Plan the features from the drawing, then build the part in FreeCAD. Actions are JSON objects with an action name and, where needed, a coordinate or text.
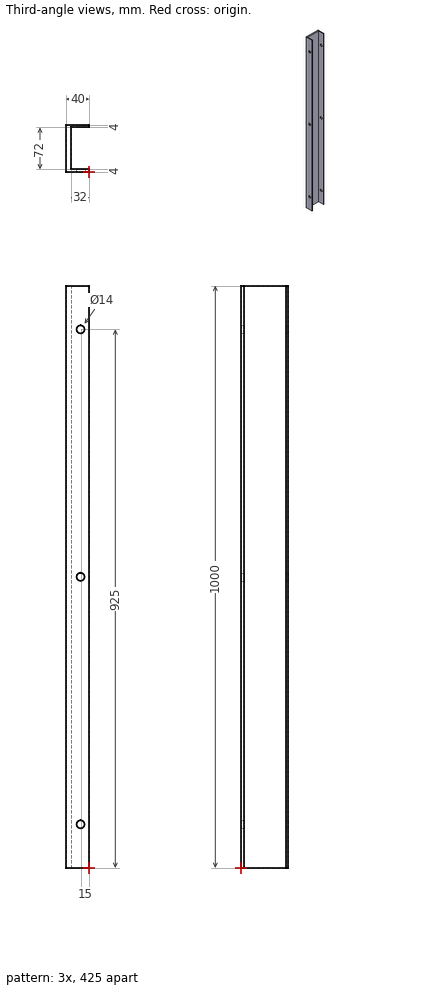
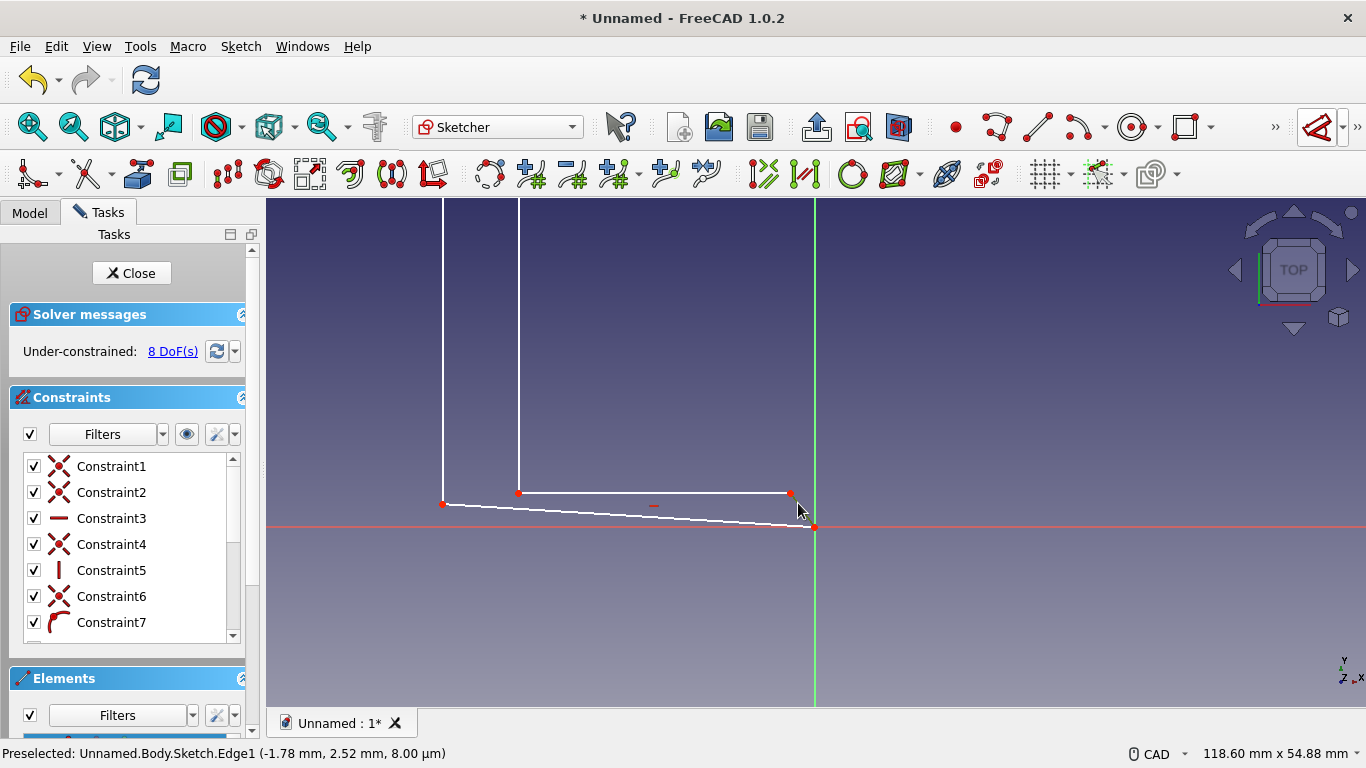
{"action": "key", "text": "v"}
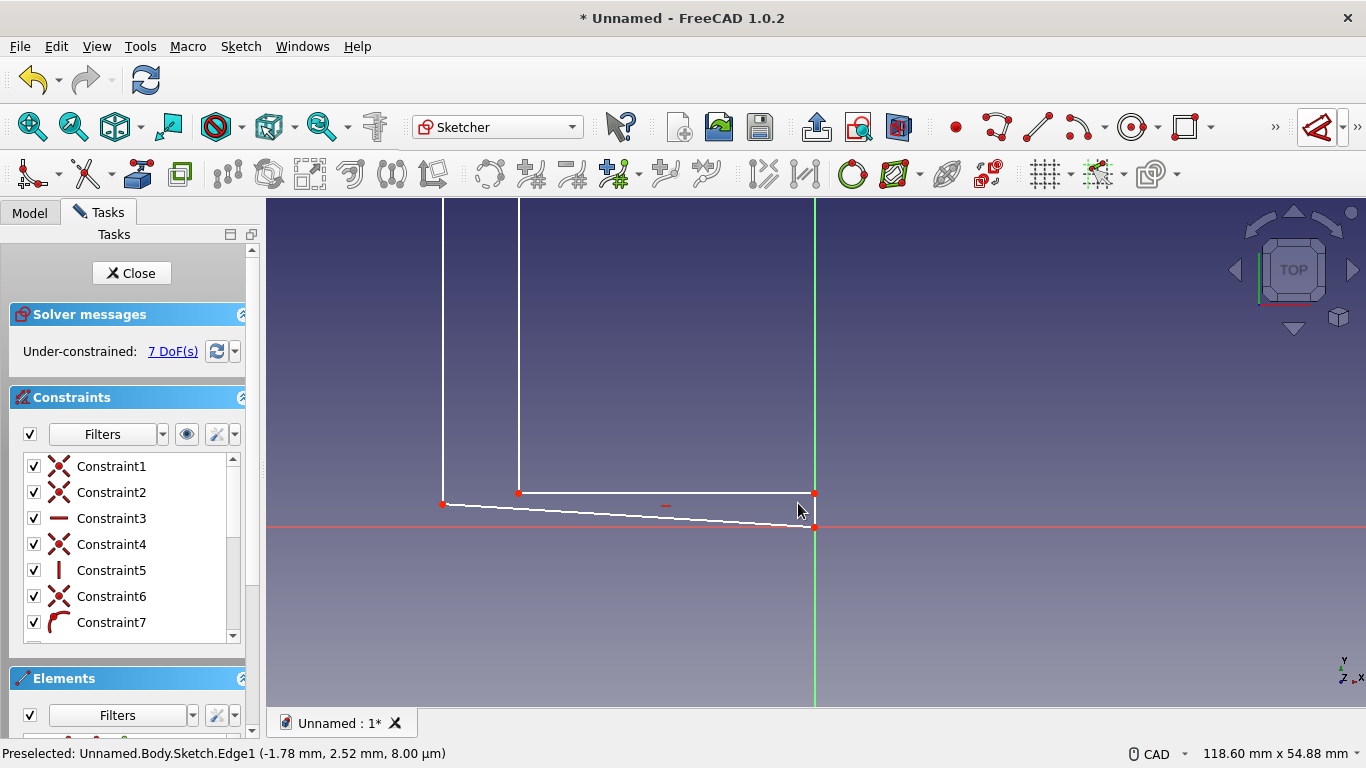
{"action": "scroll", "coordinate": [844, 679], "scroll_direction": "down", "scroll_amount": 4}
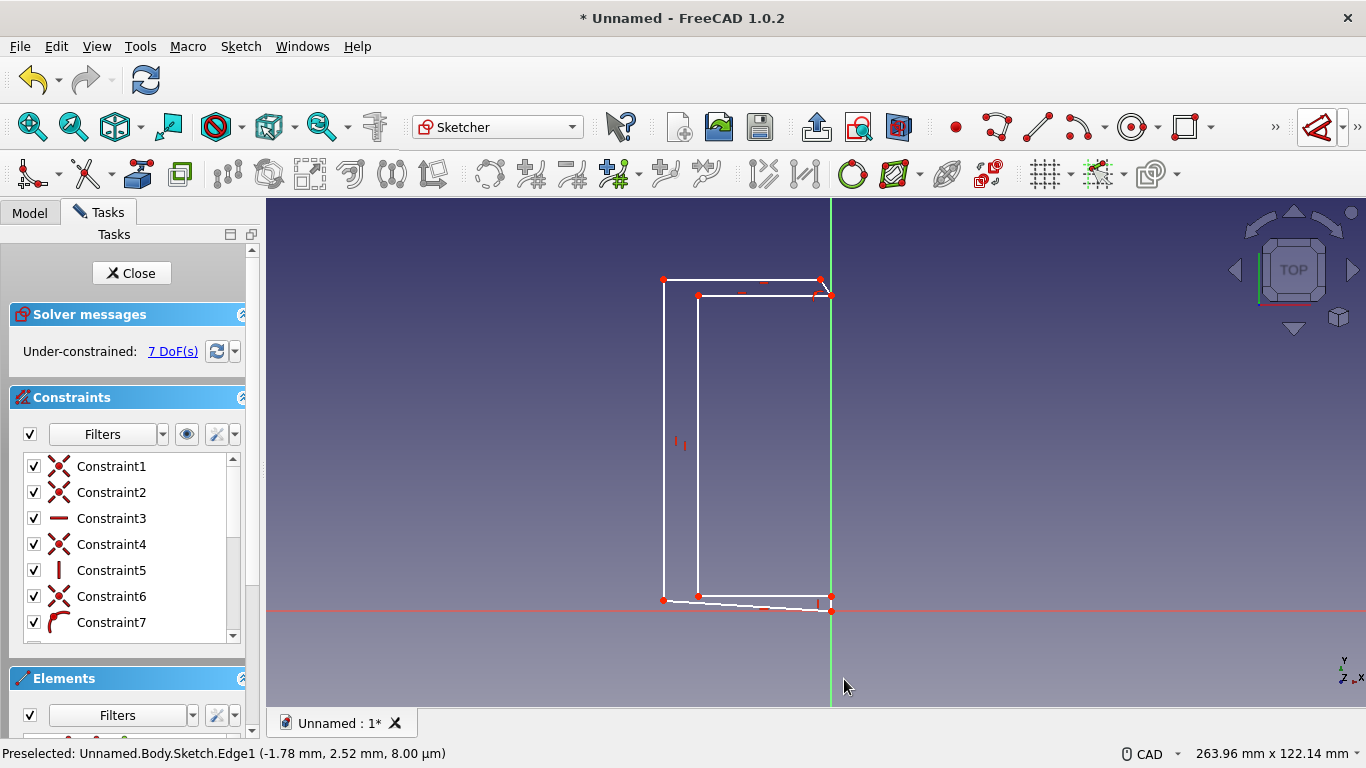
{"action": "scroll", "coordinate": [824, 284], "scroll_direction": "up", "scroll_amount": 5}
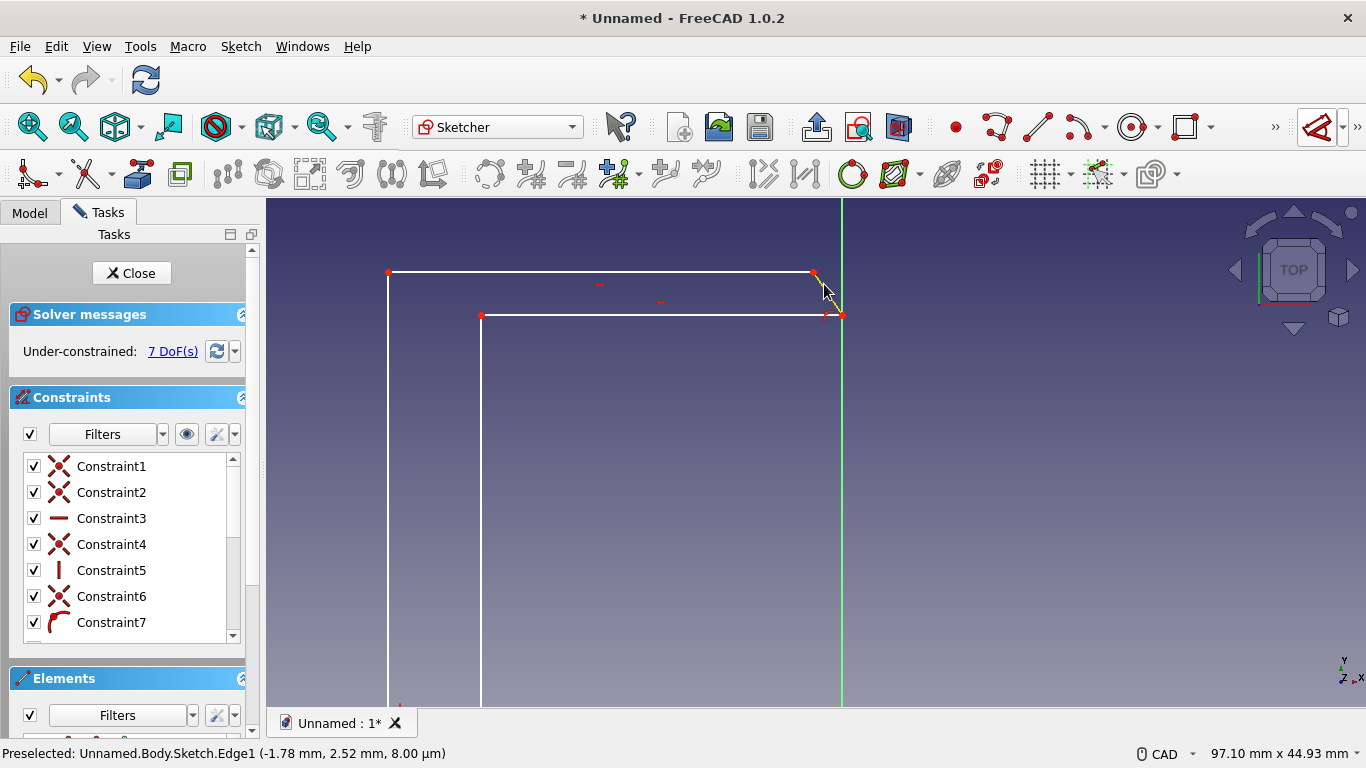
{"action": "left_click", "coordinate": [822, 285]}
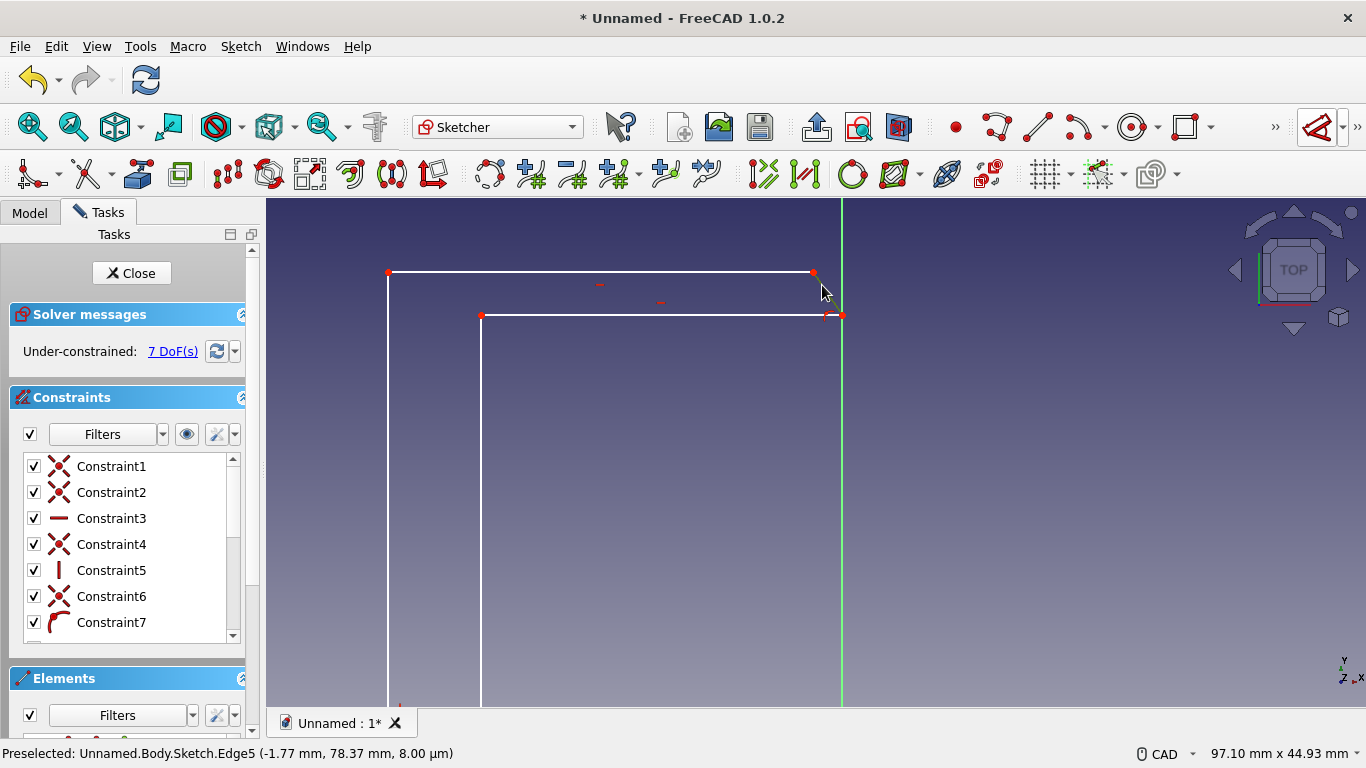
{"action": "key", "text": "v"}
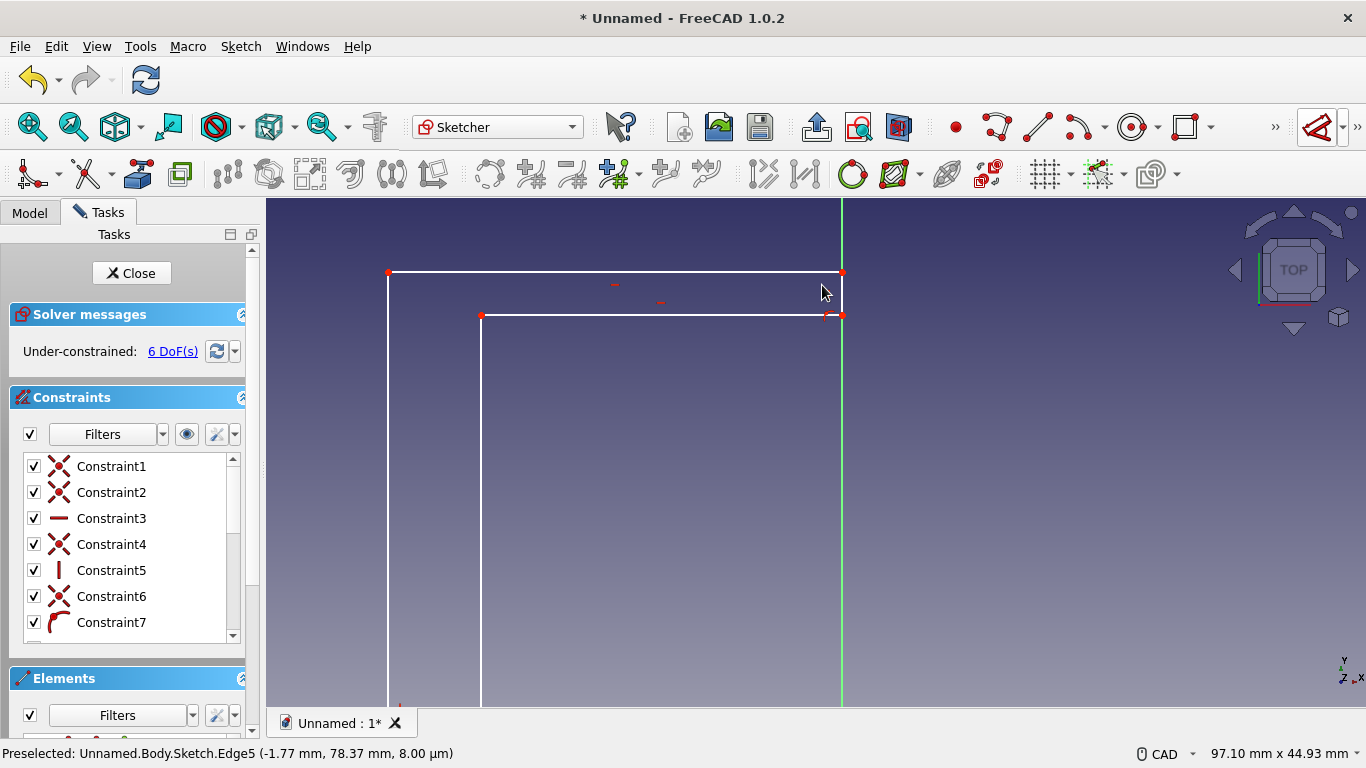
{"action": "scroll", "coordinate": [824, 297], "scroll_direction": "down", "scroll_amount": 5}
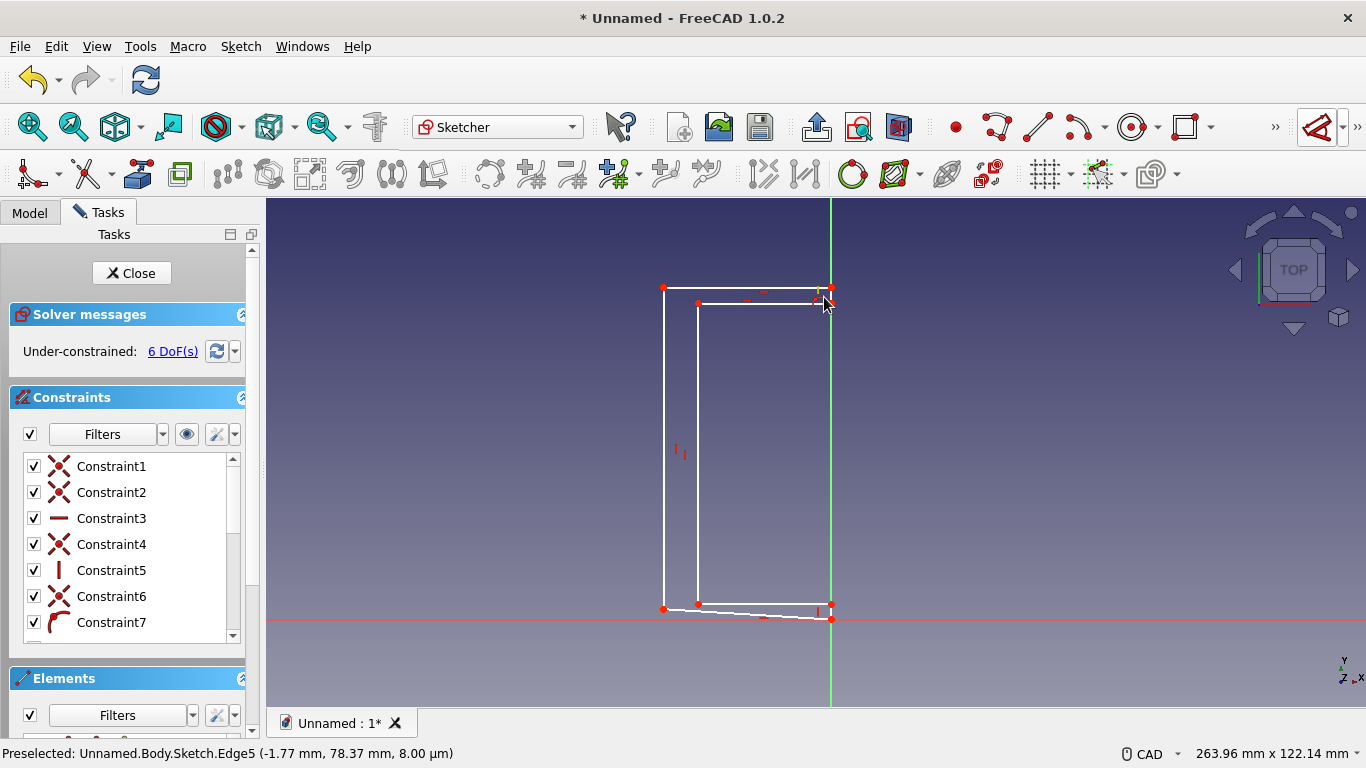
{"action": "scroll", "coordinate": [714, 612], "scroll_direction": "up", "scroll_amount": 4}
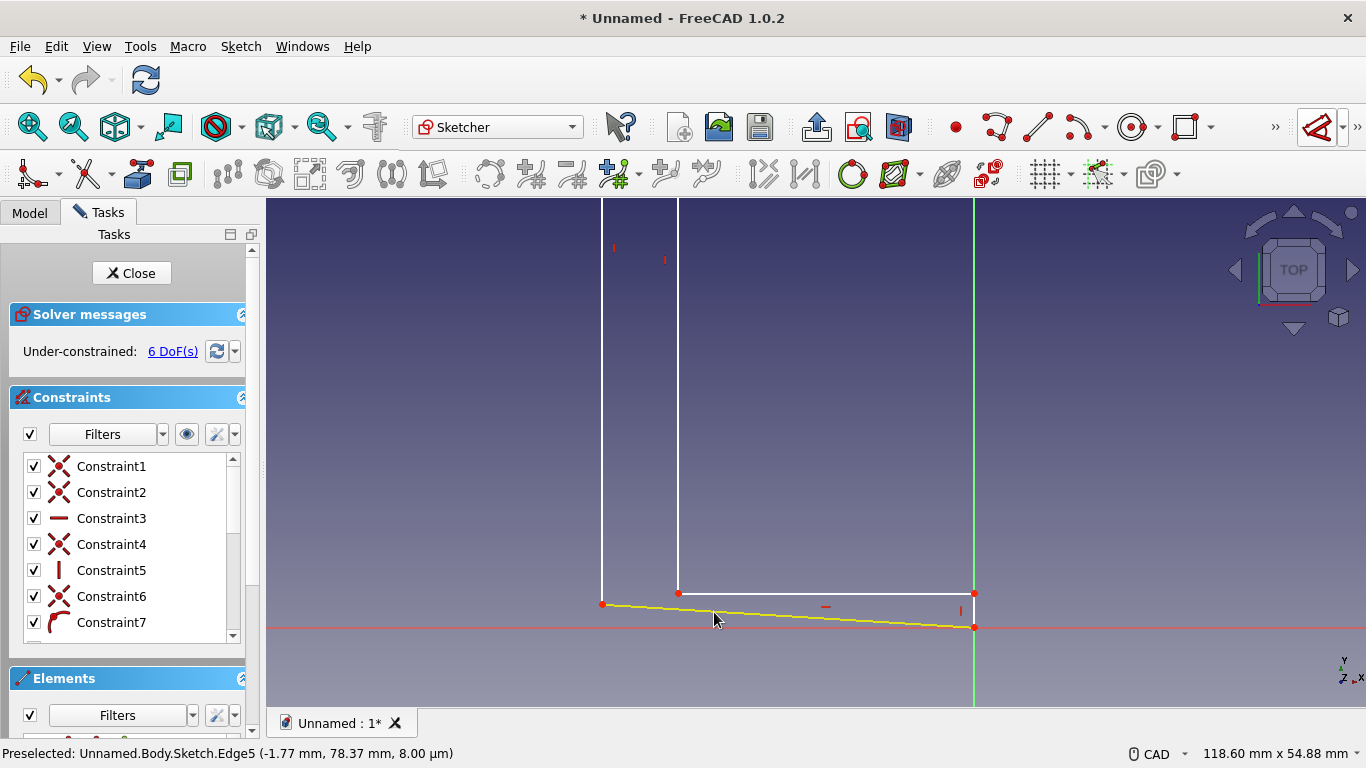
{"action": "left_click", "coordinate": [714, 612]}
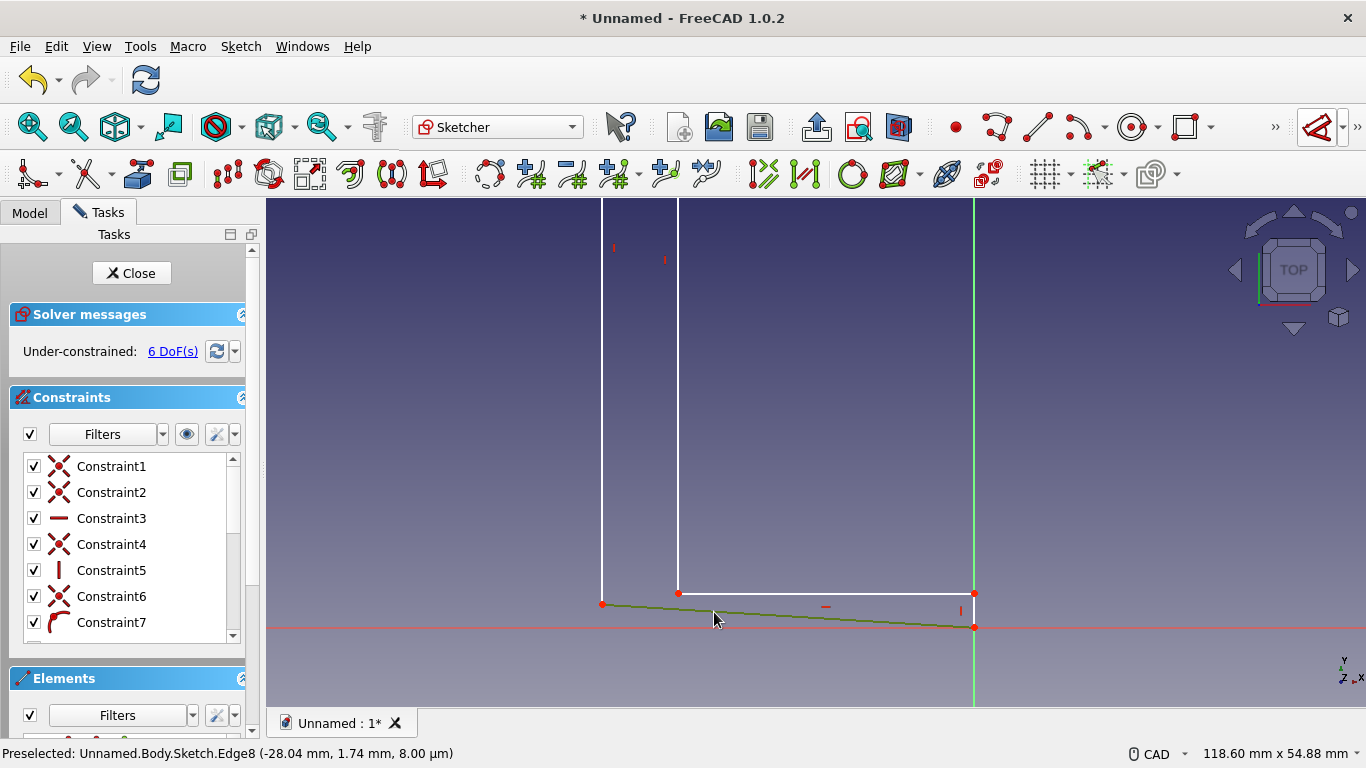
{"action": "key", "text": "h"}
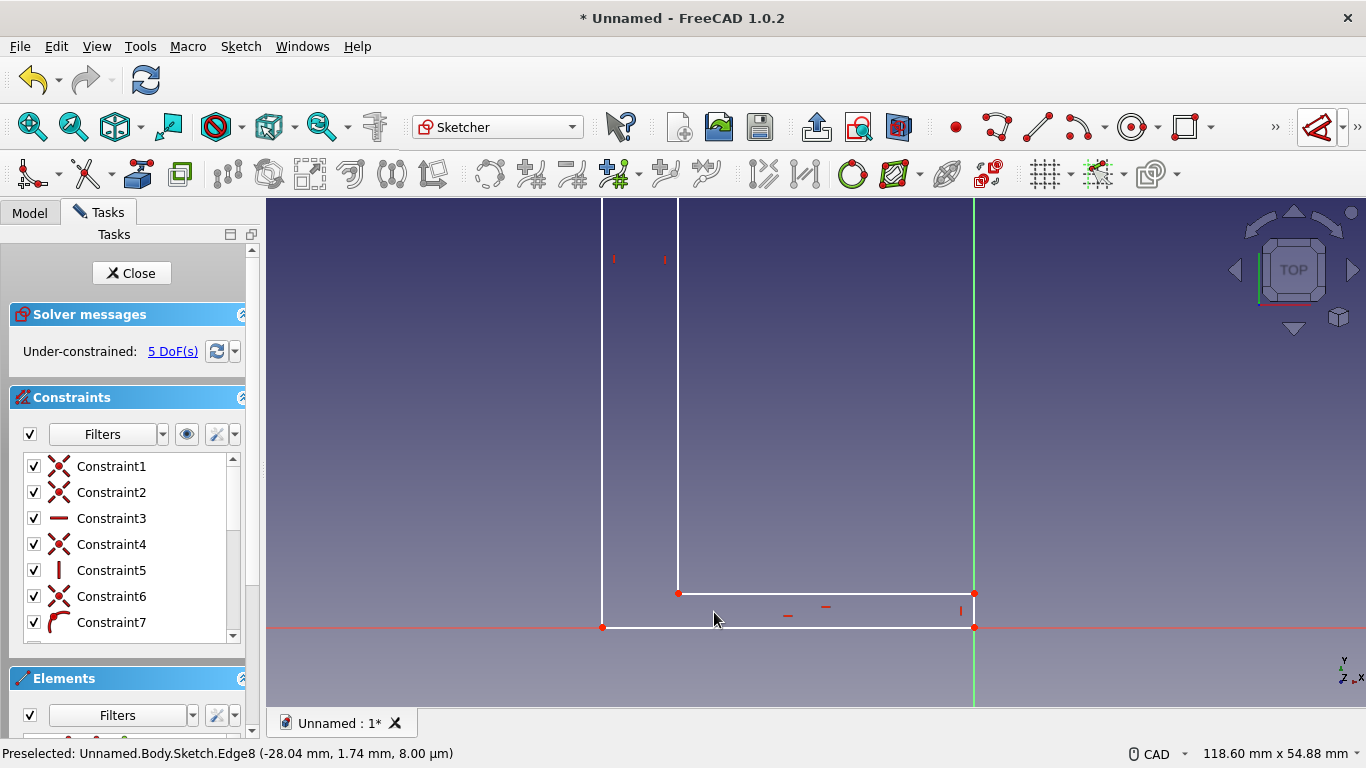
{"action": "left_click", "coordinate": [1316, 128]}